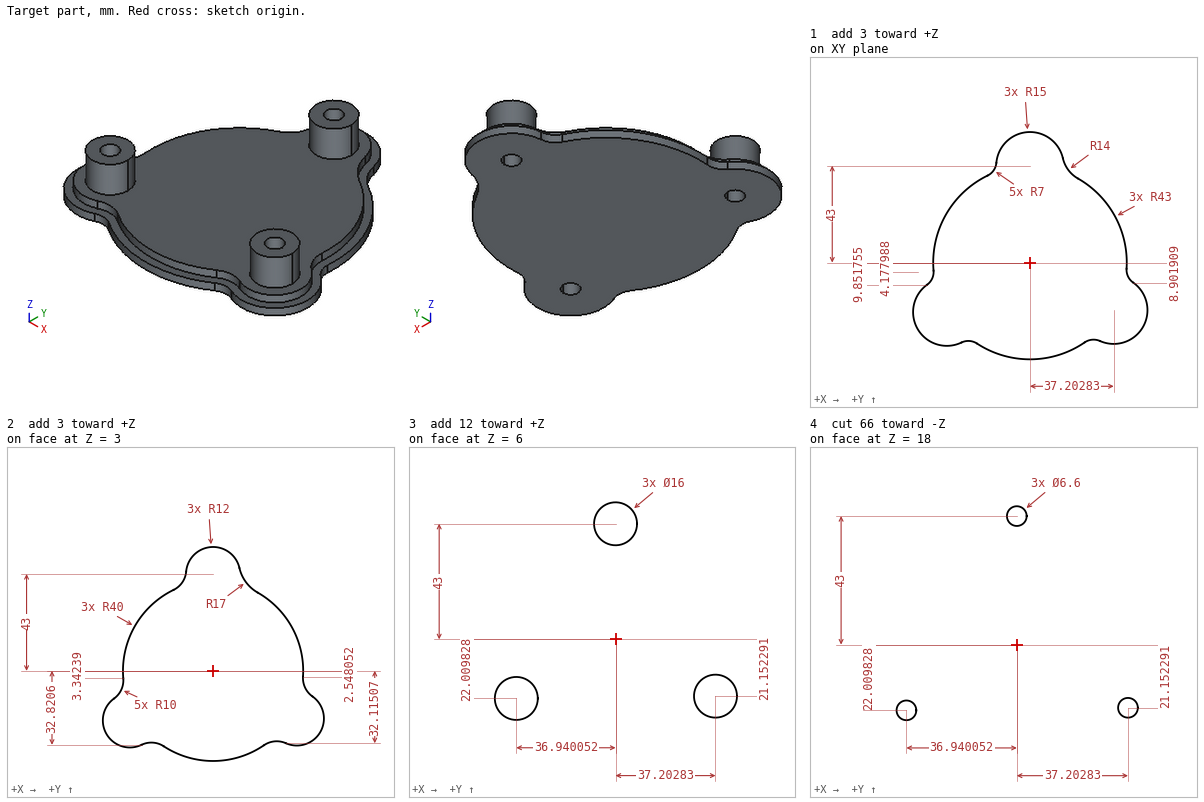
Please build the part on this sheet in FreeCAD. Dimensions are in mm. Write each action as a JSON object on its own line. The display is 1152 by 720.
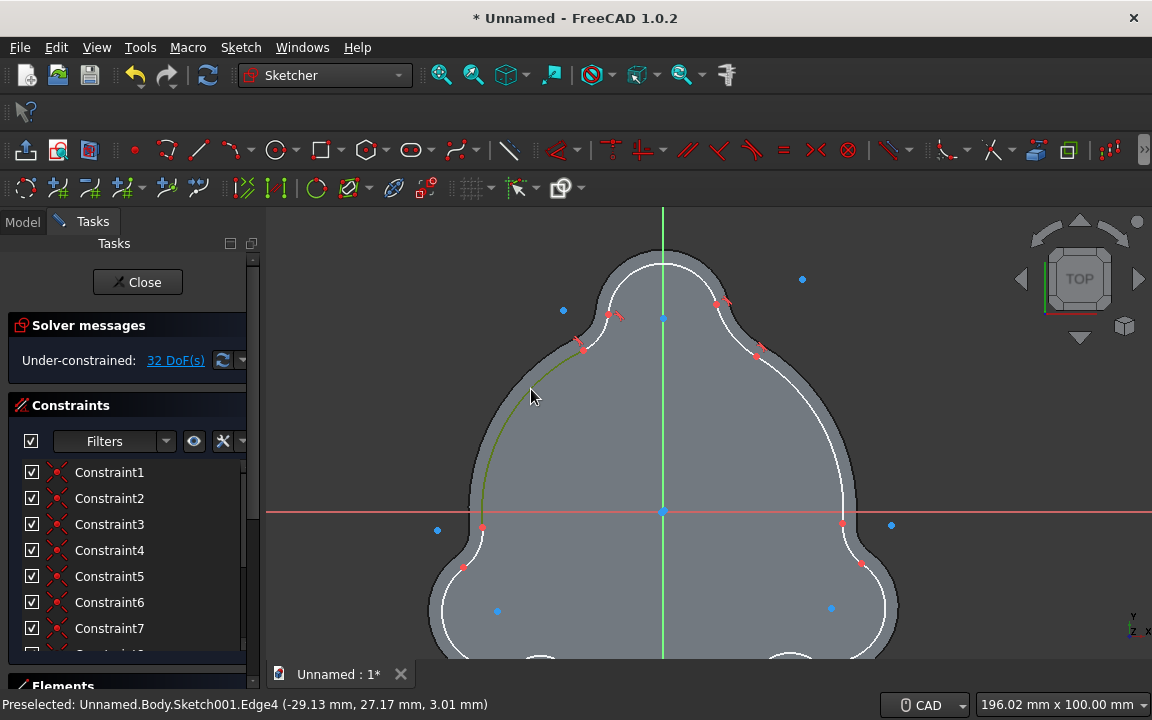
{"action": "left_click", "coordinate": [474, 558]}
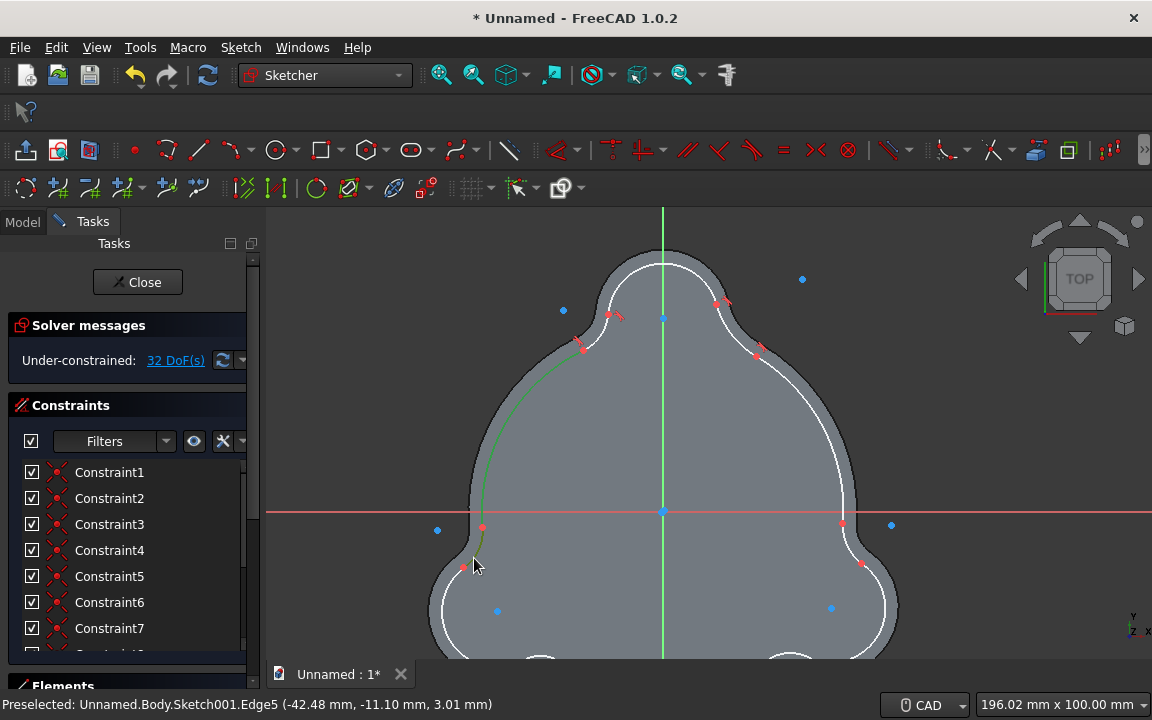
{"action": "left_click", "coordinate": [752, 150]}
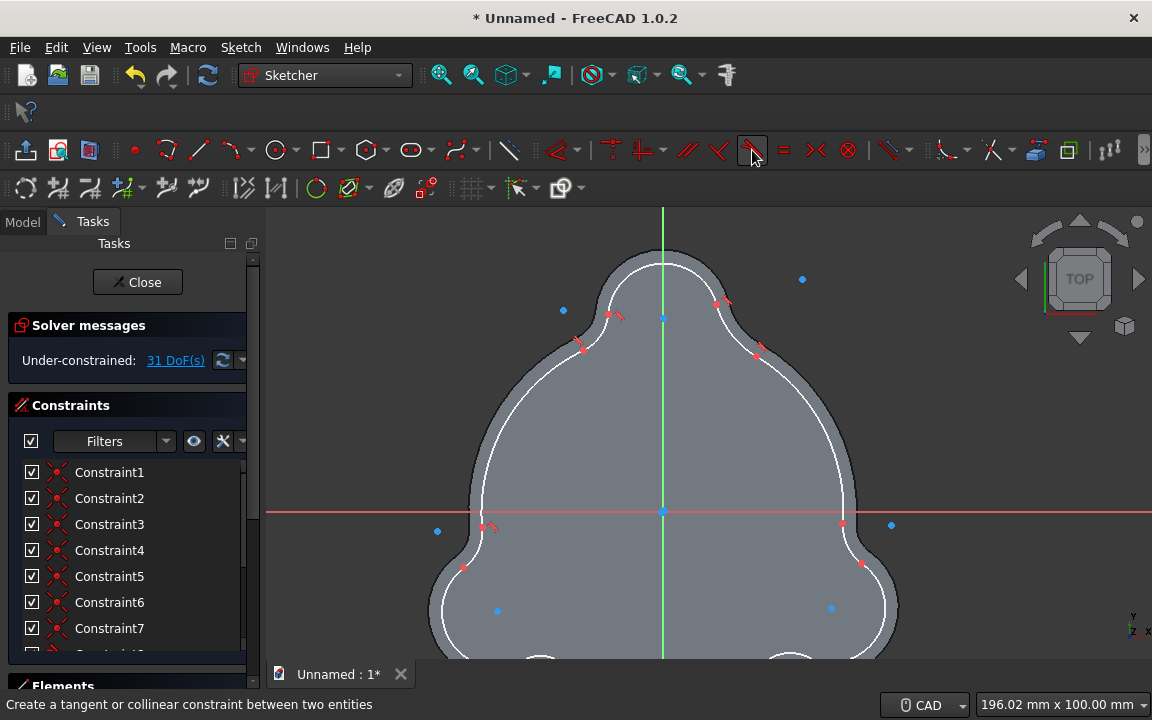
{"action": "left_click", "coordinate": [474, 558]}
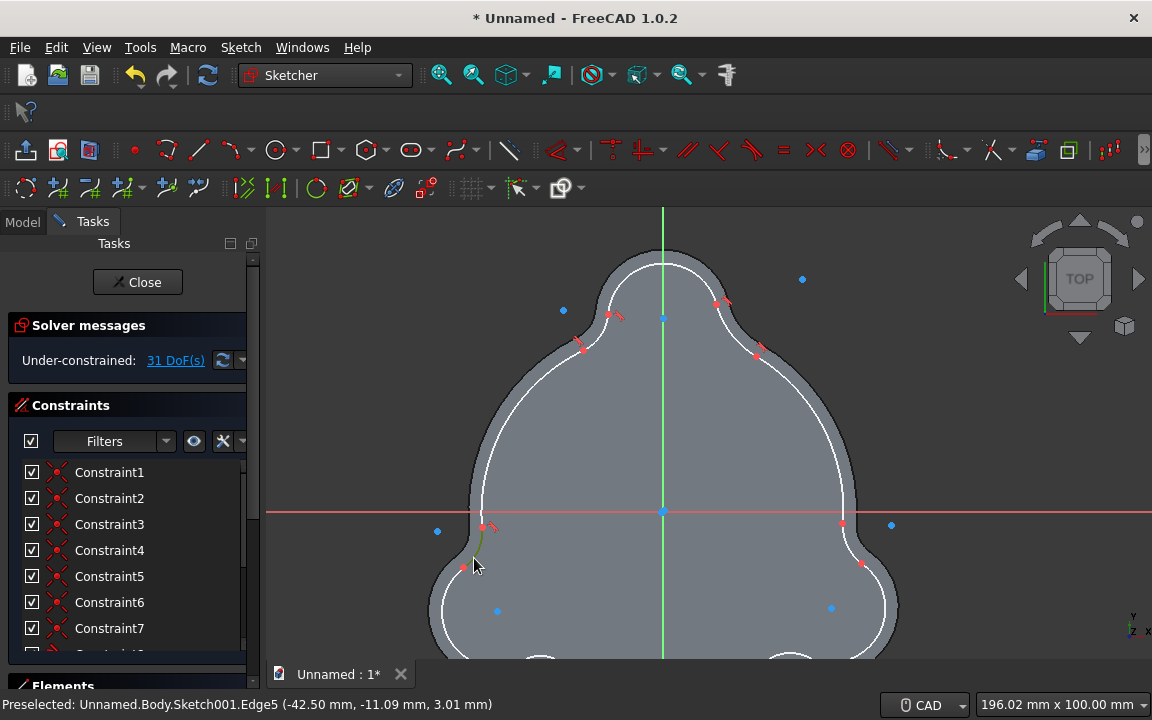
{"action": "left_click", "coordinate": [442, 609]}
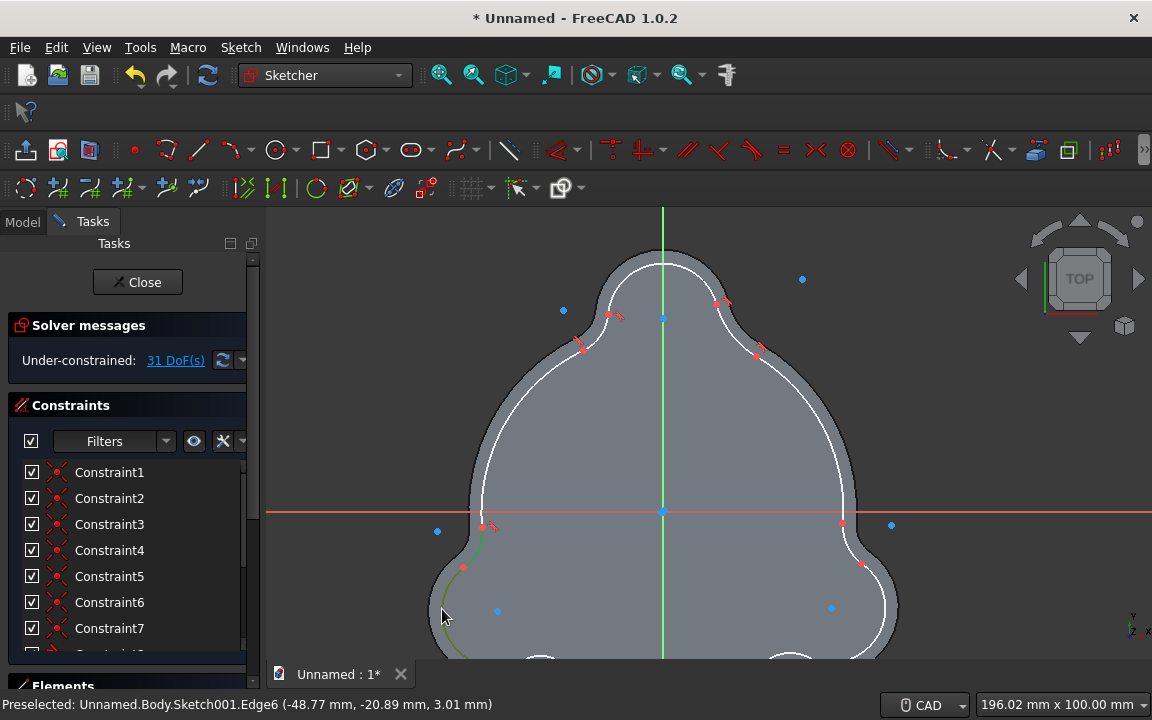
{"action": "left_click", "coordinate": [752, 150]}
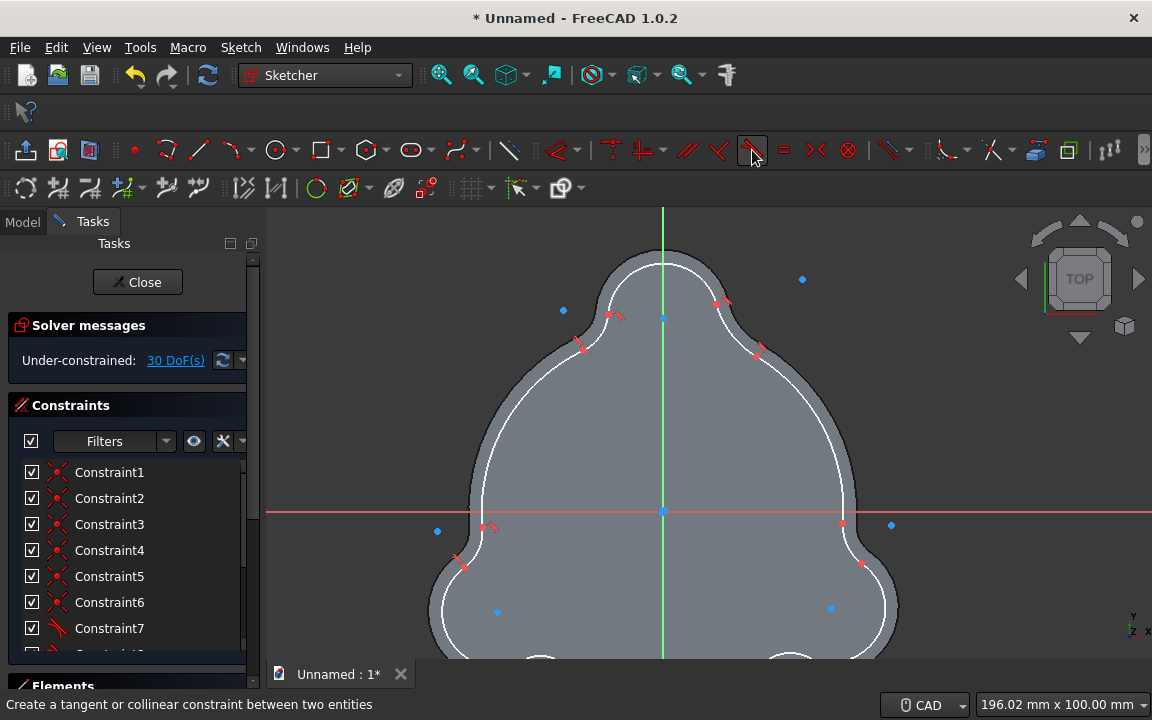
{"action": "left_click", "coordinate": [442, 609]}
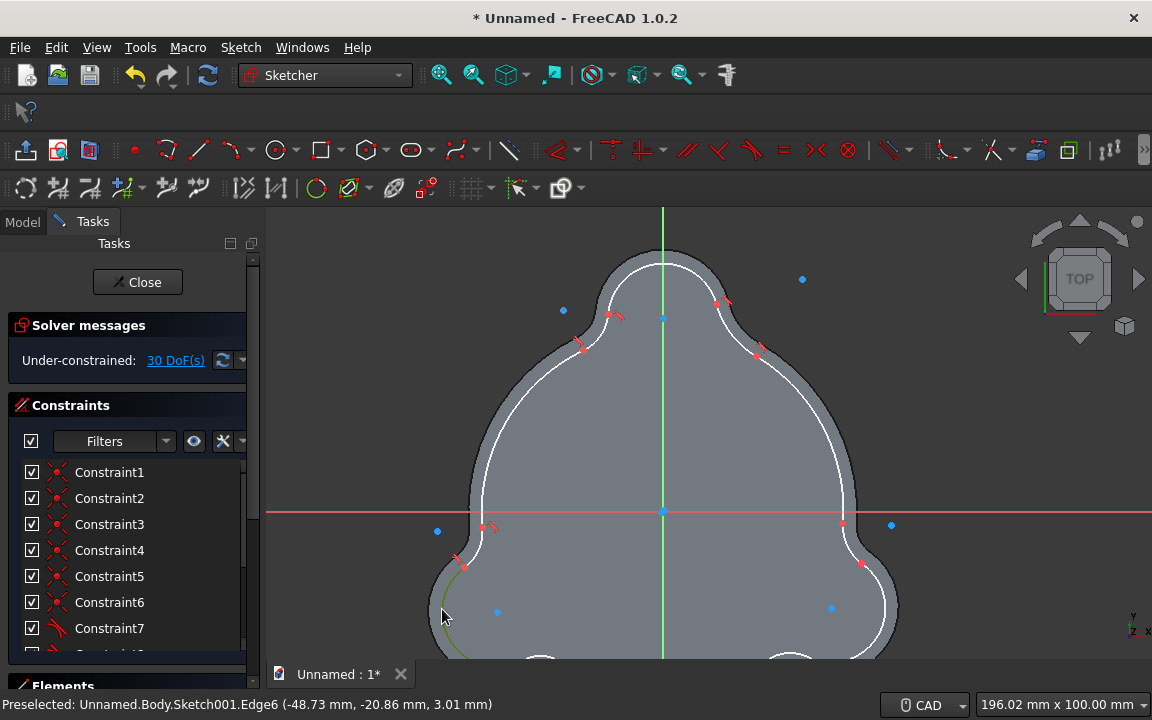
{"action": "scroll", "coordinate": [593, 342], "scroll_direction": "down", "scroll_amount": 2}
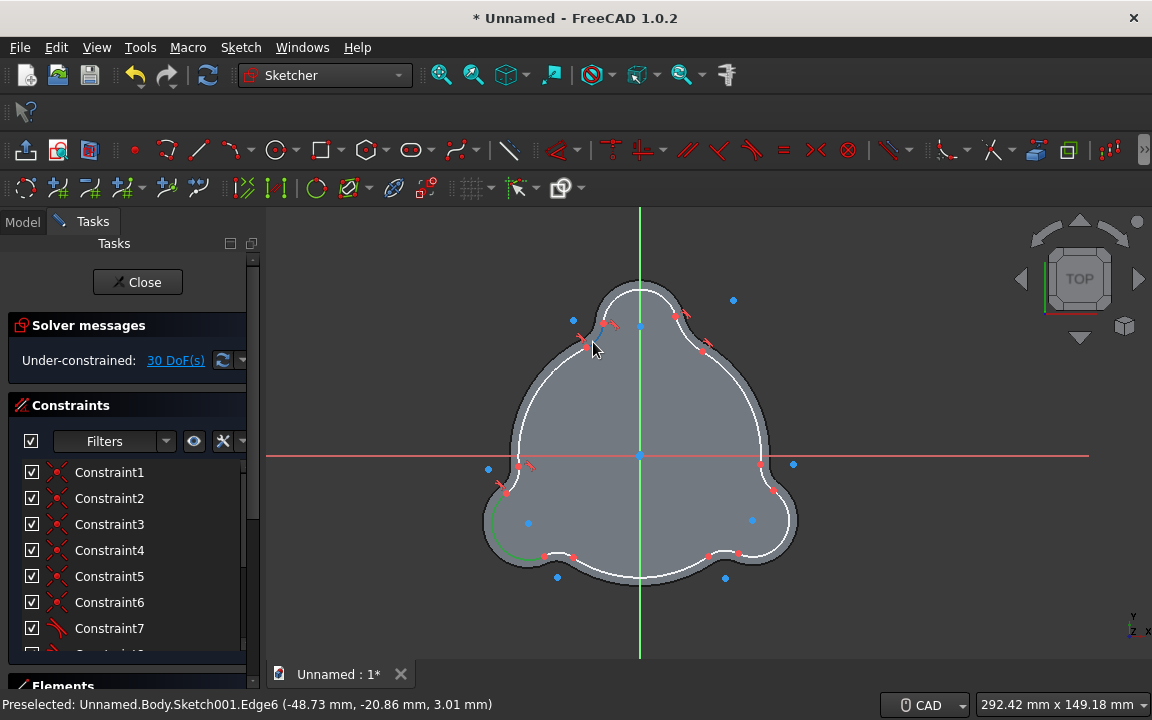
{"action": "scroll", "coordinate": [565, 554], "scroll_direction": "up", "scroll_amount": 3}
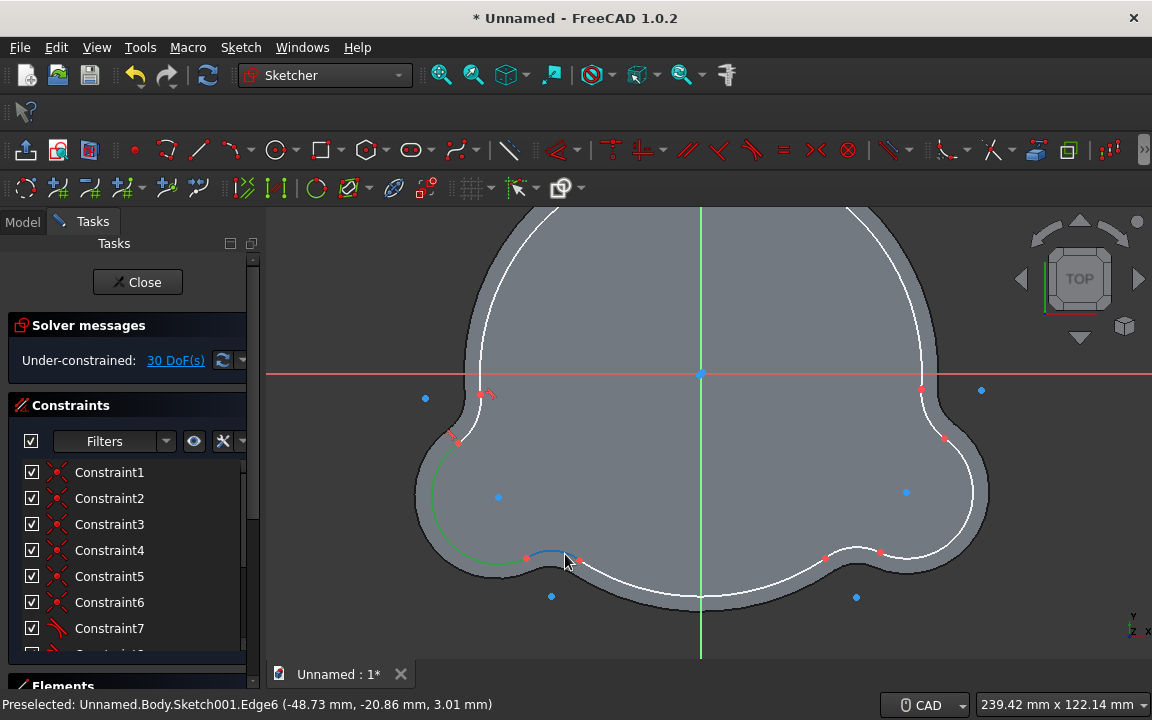
{"action": "left_click", "coordinate": [564, 553]}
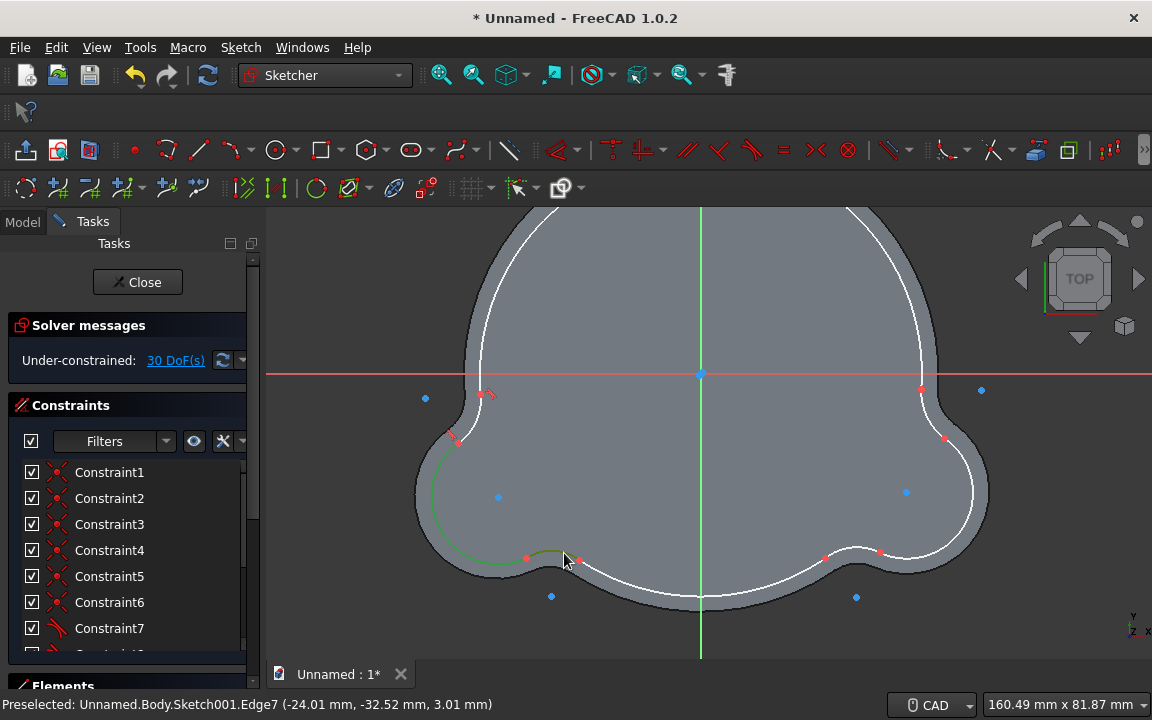
{"action": "key", "text": "t"}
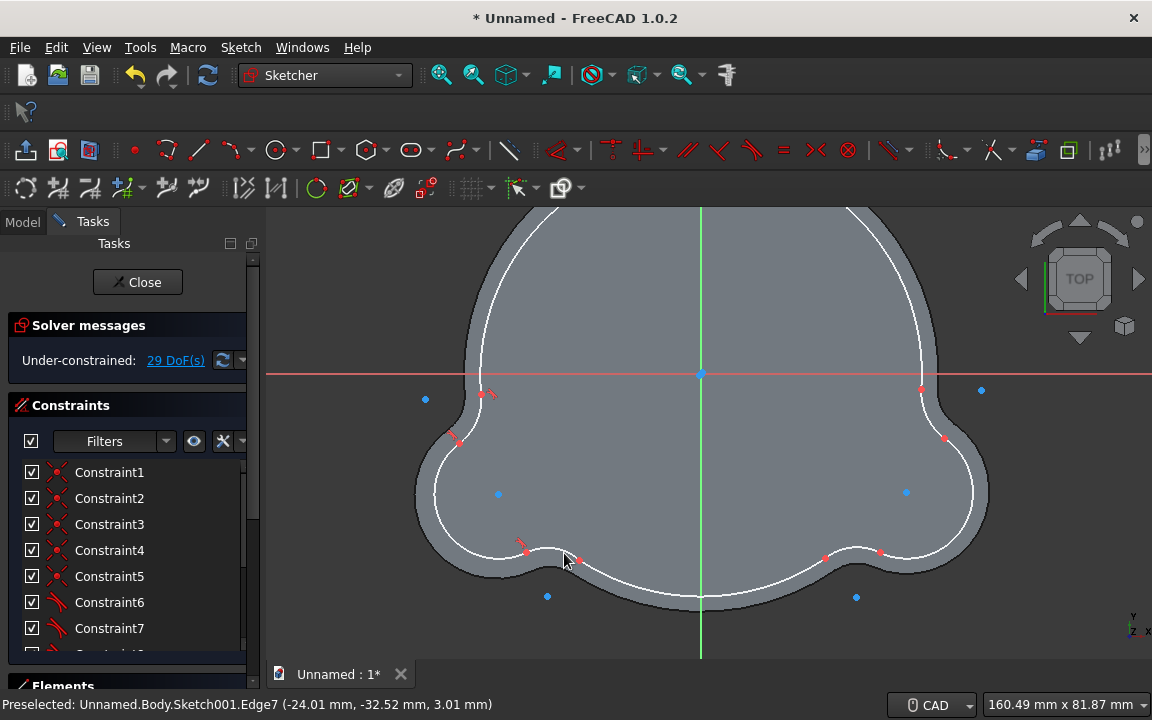
{"action": "left_click", "coordinate": [565, 551]}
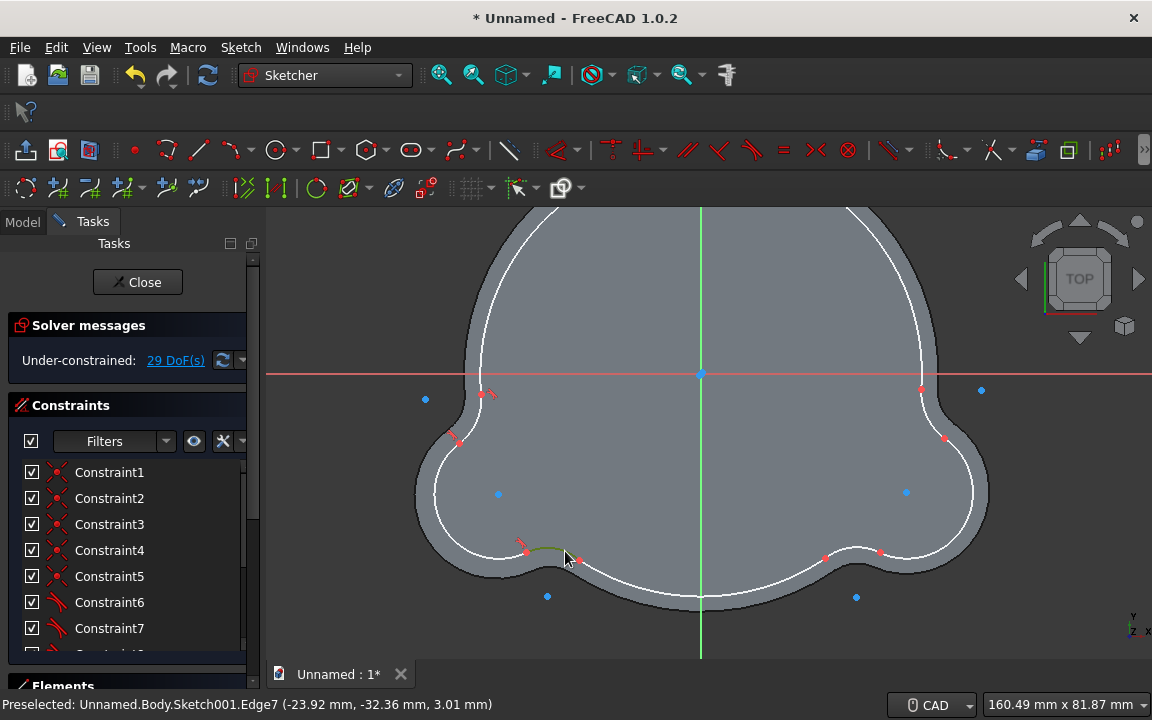
{"action": "left_click", "coordinate": [651, 591]}